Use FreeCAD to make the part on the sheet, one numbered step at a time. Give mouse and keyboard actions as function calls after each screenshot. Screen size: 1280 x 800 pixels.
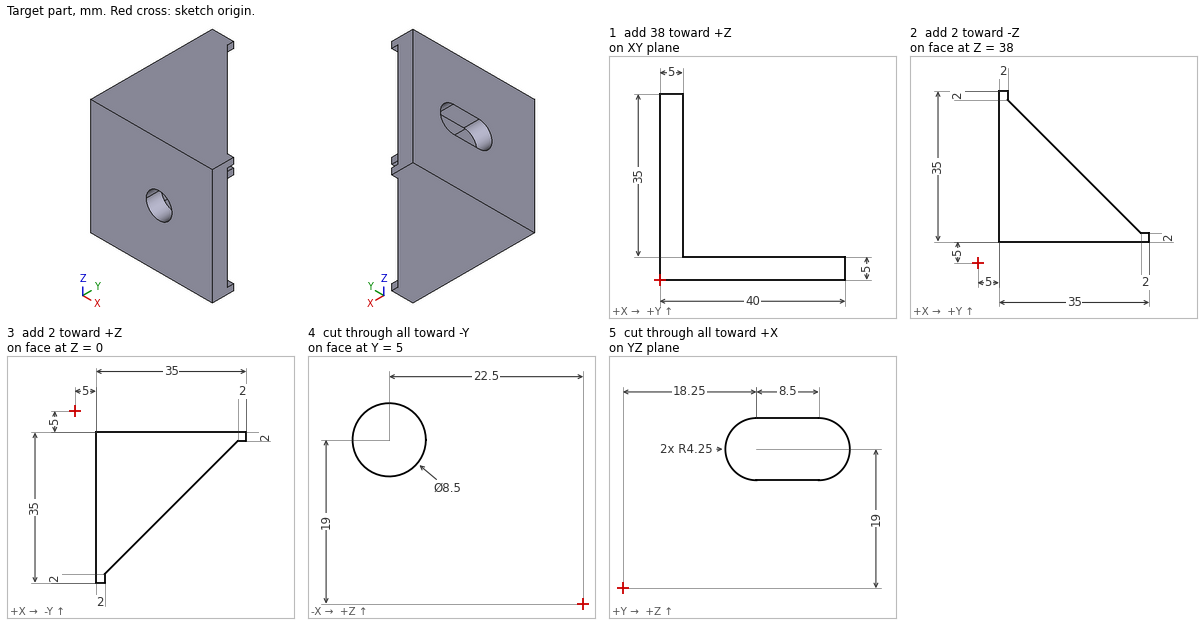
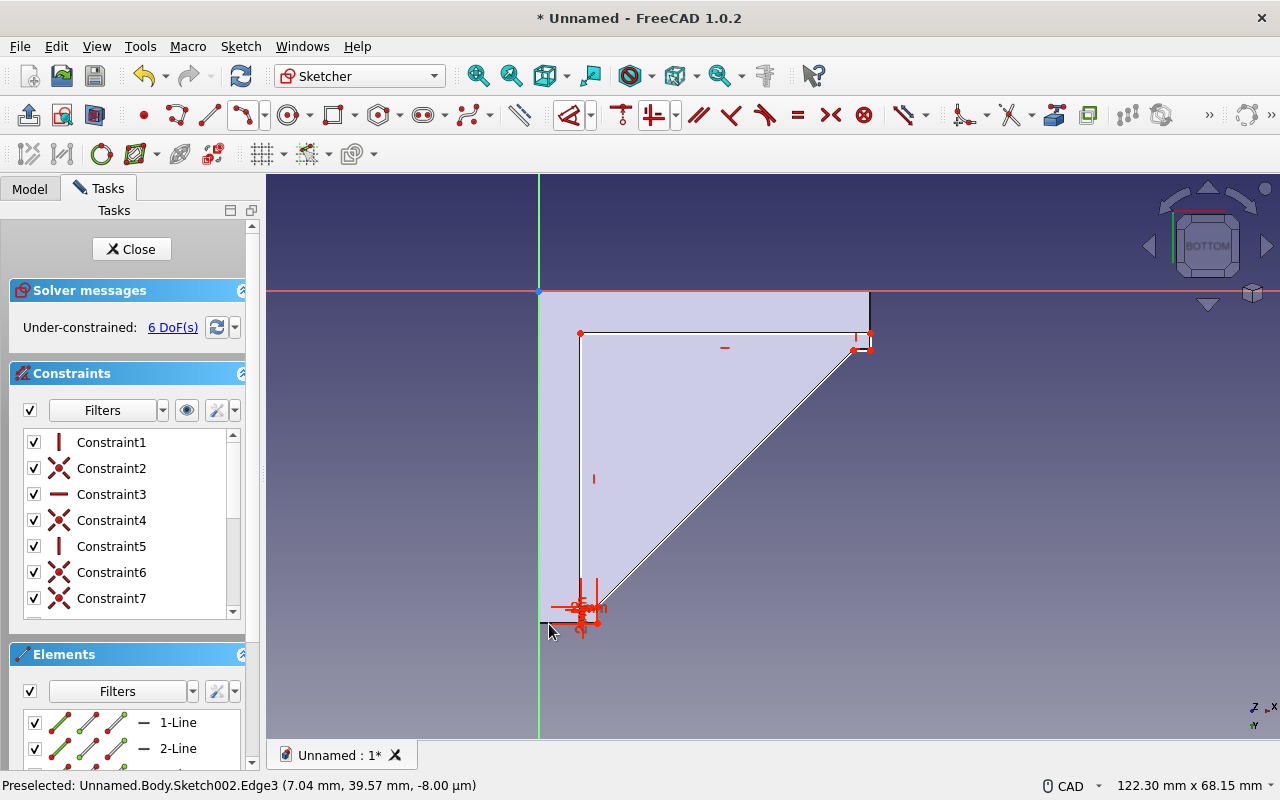
scroll(859, 351, up, 5)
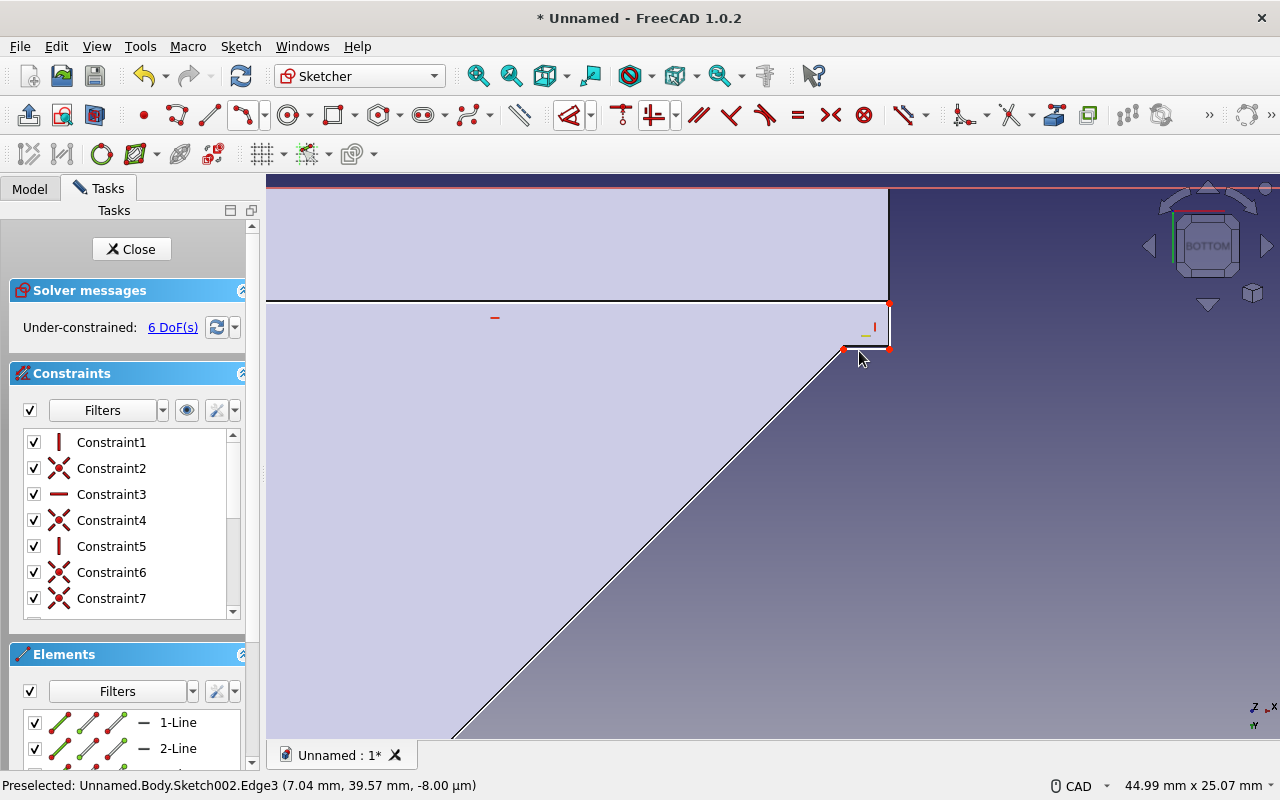
click(857, 349)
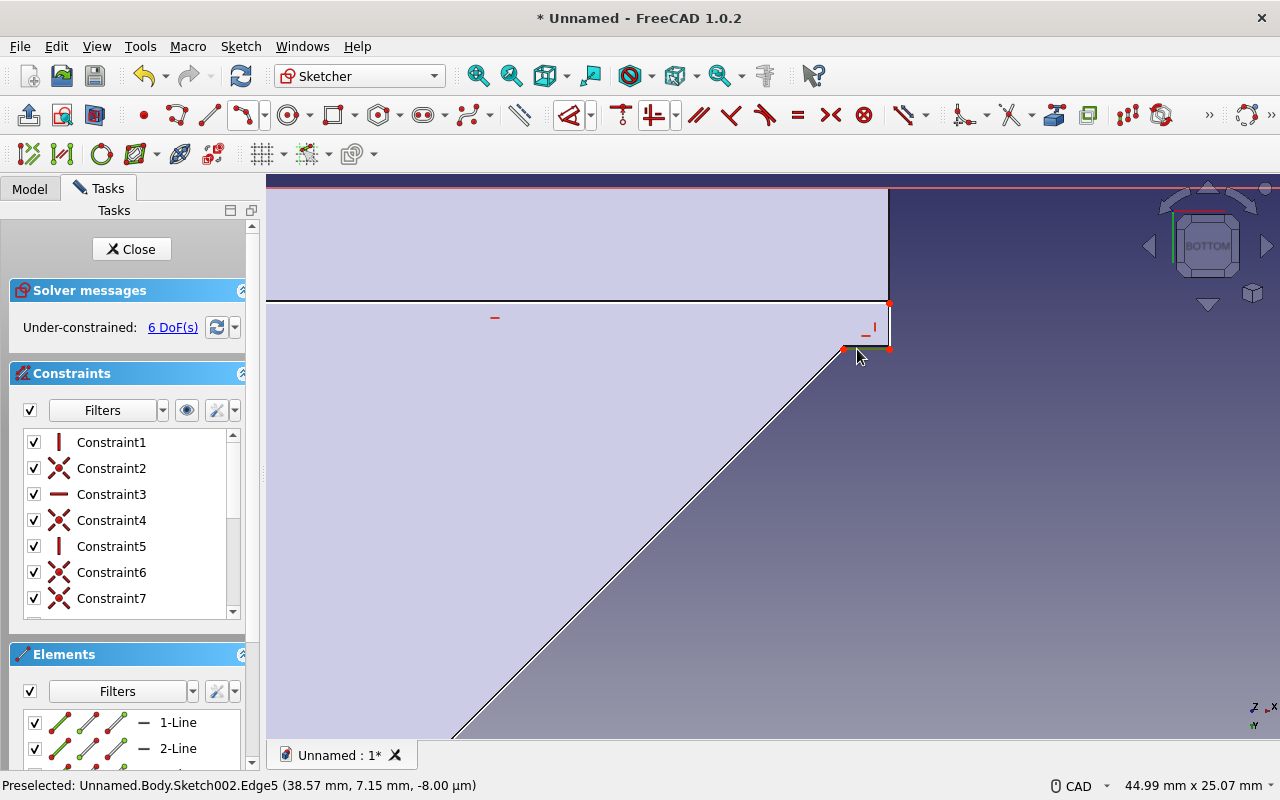
key(l)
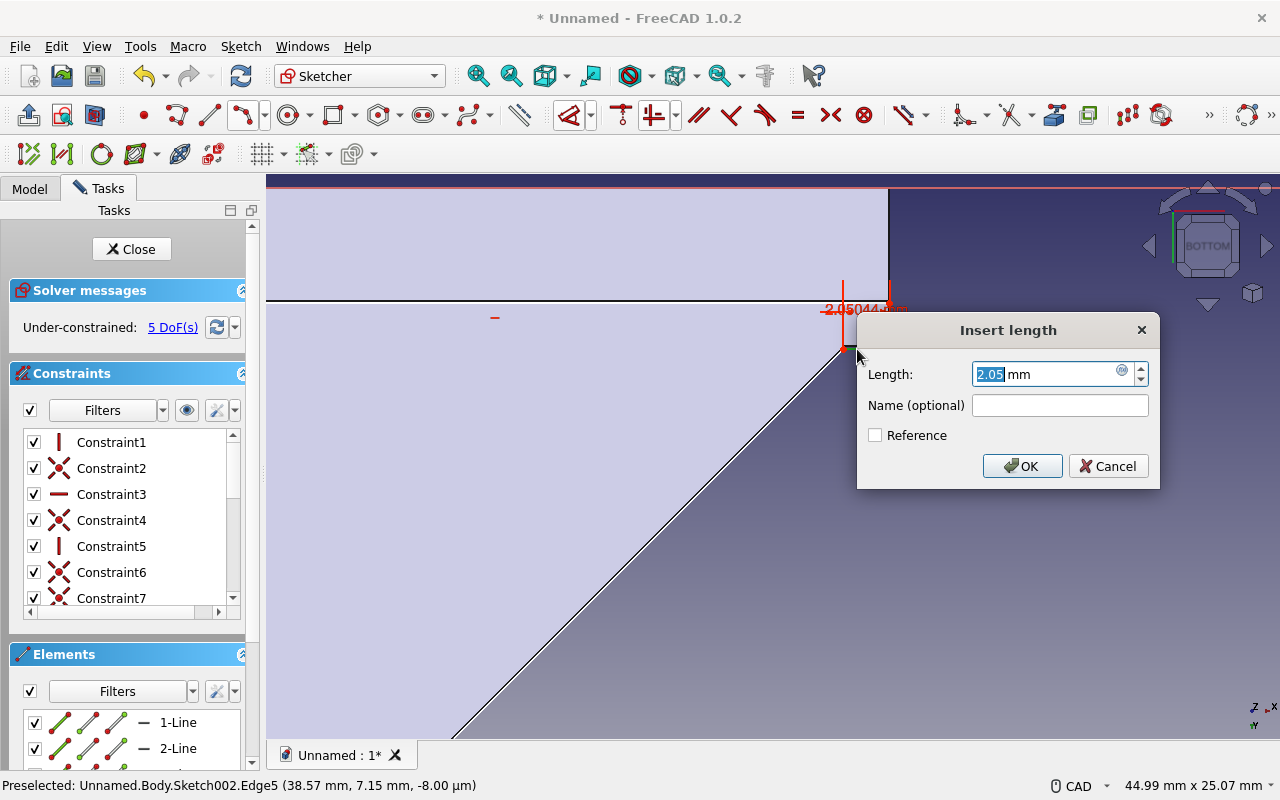
text(2)
key(Return)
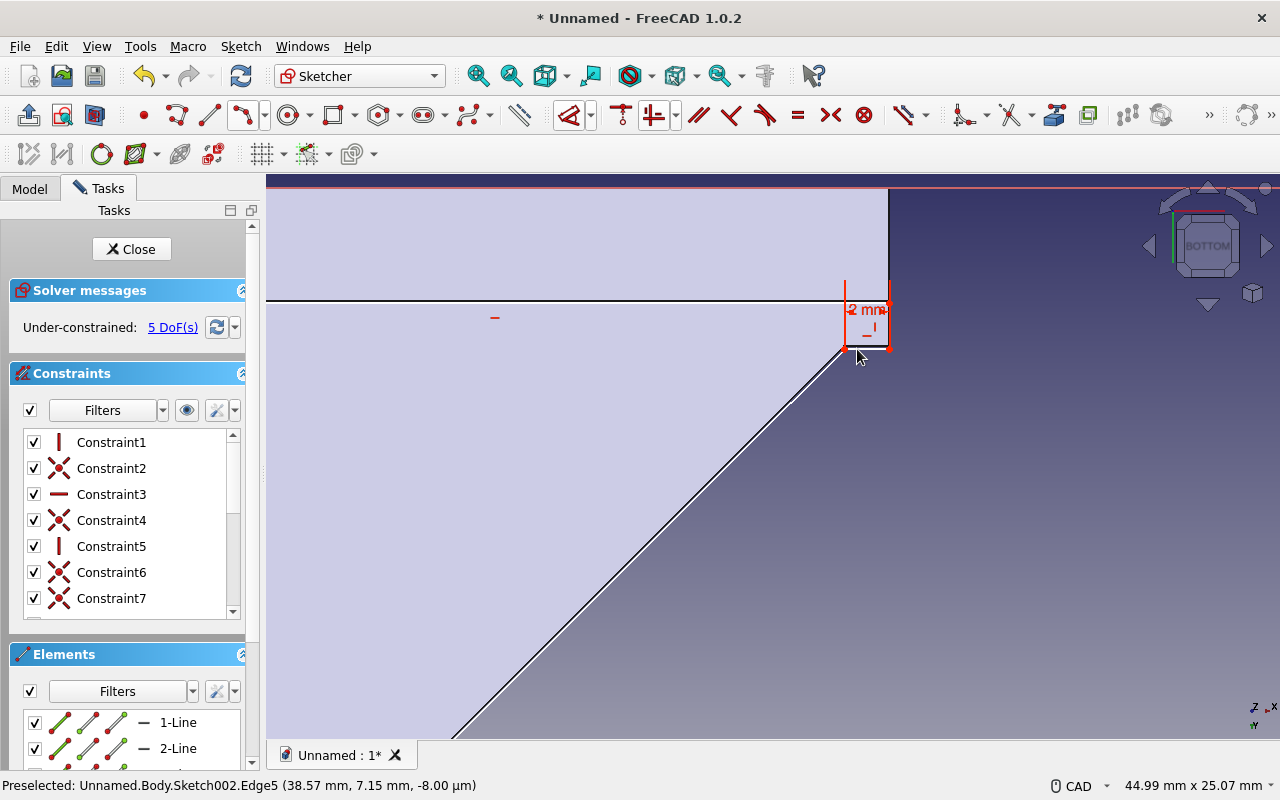
click(890, 336)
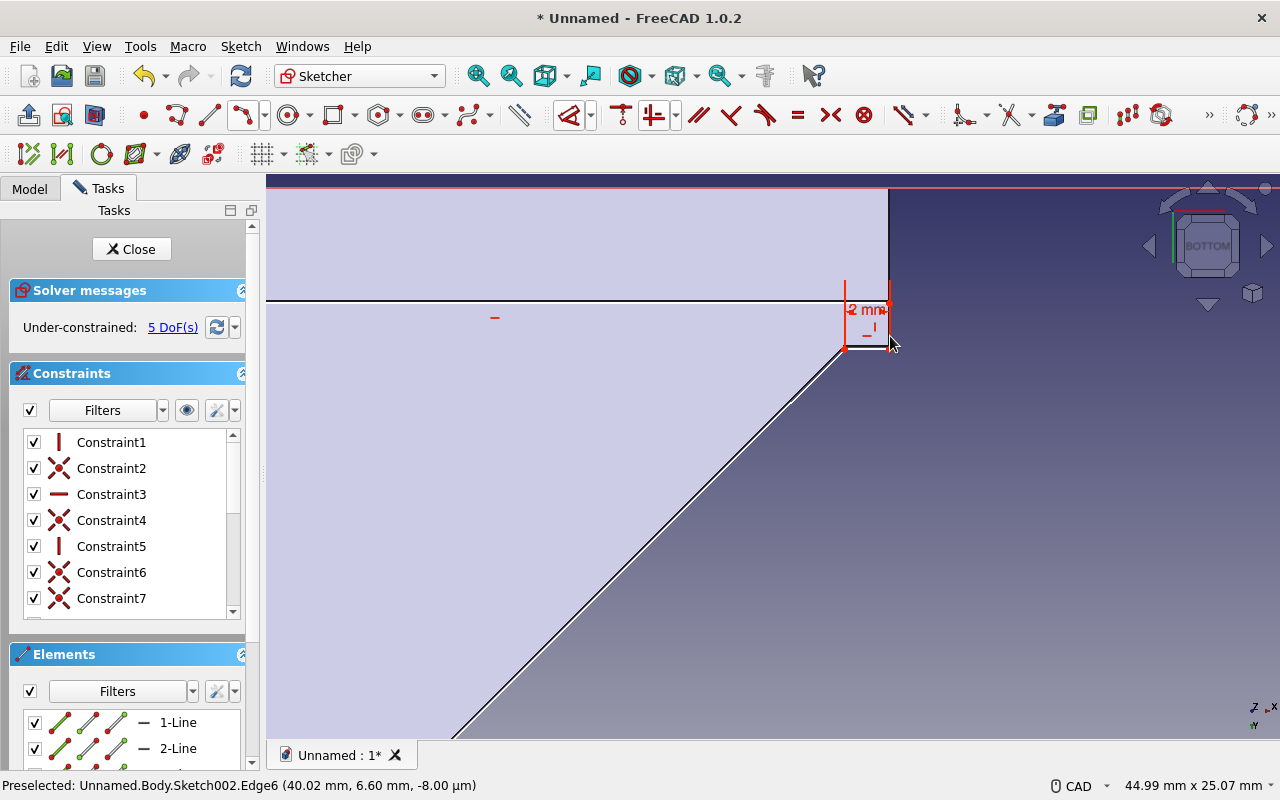
click(590, 116)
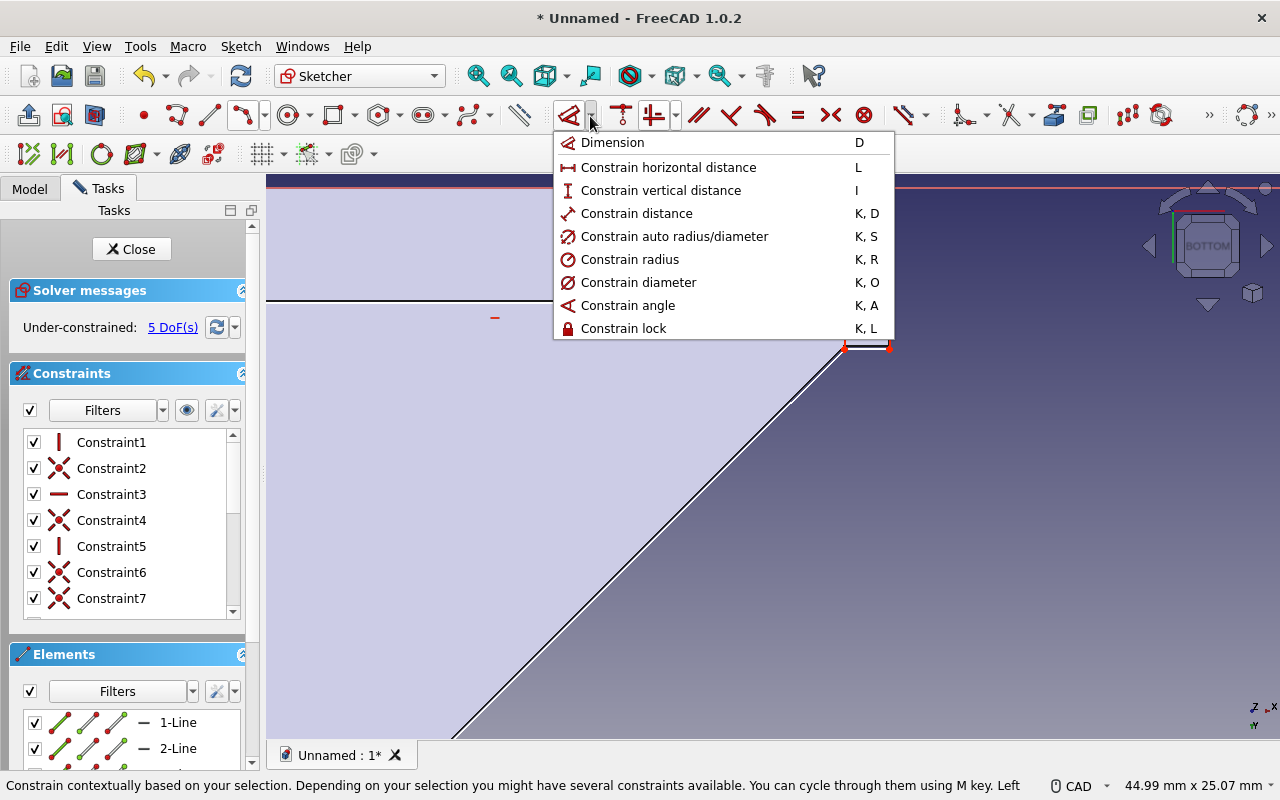
click(724, 190)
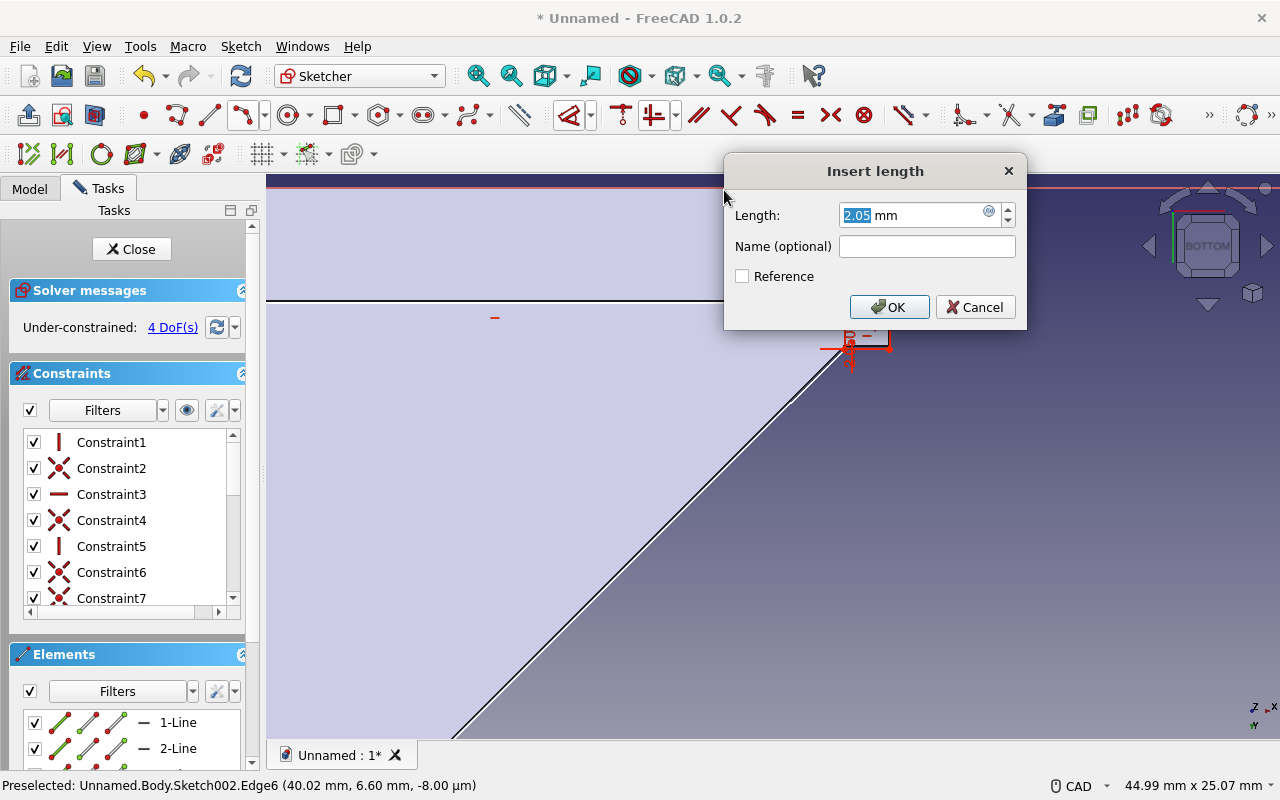
text(2)
key(Return)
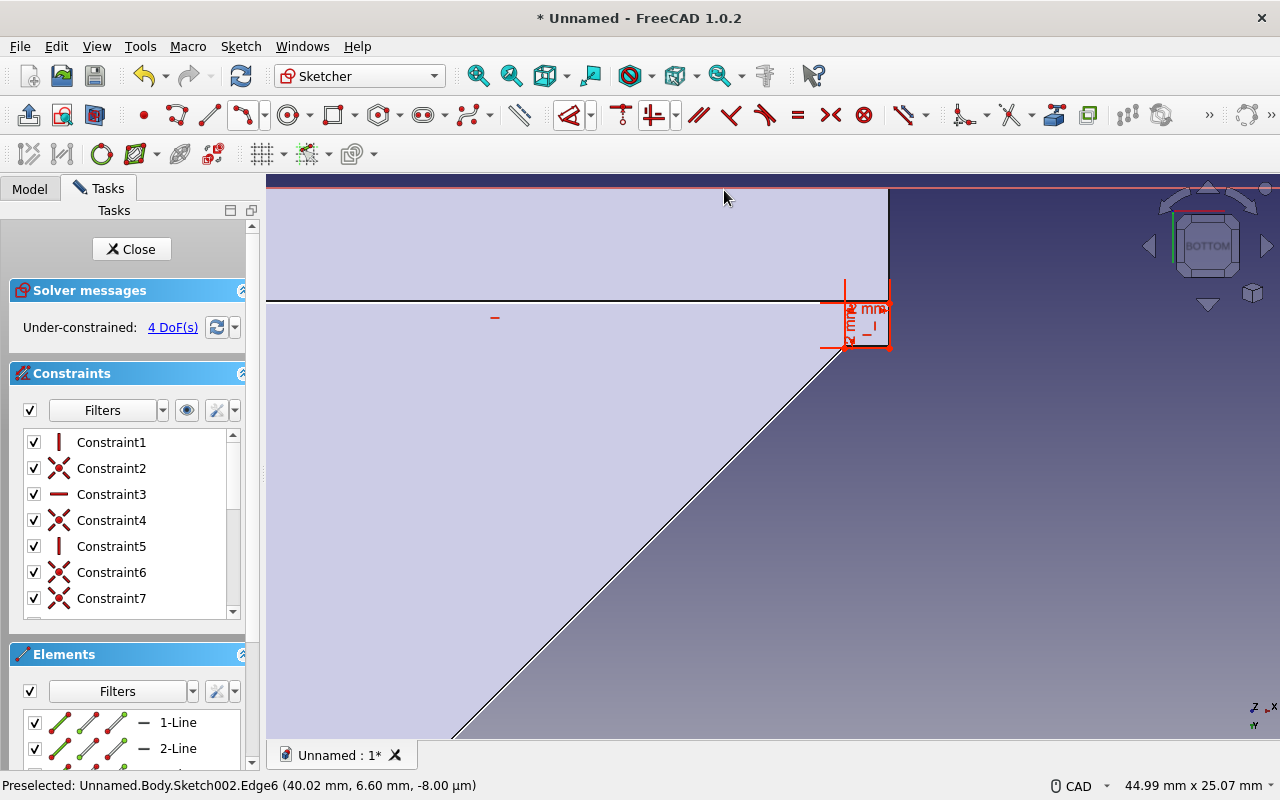
scroll(859, 350, down, 5)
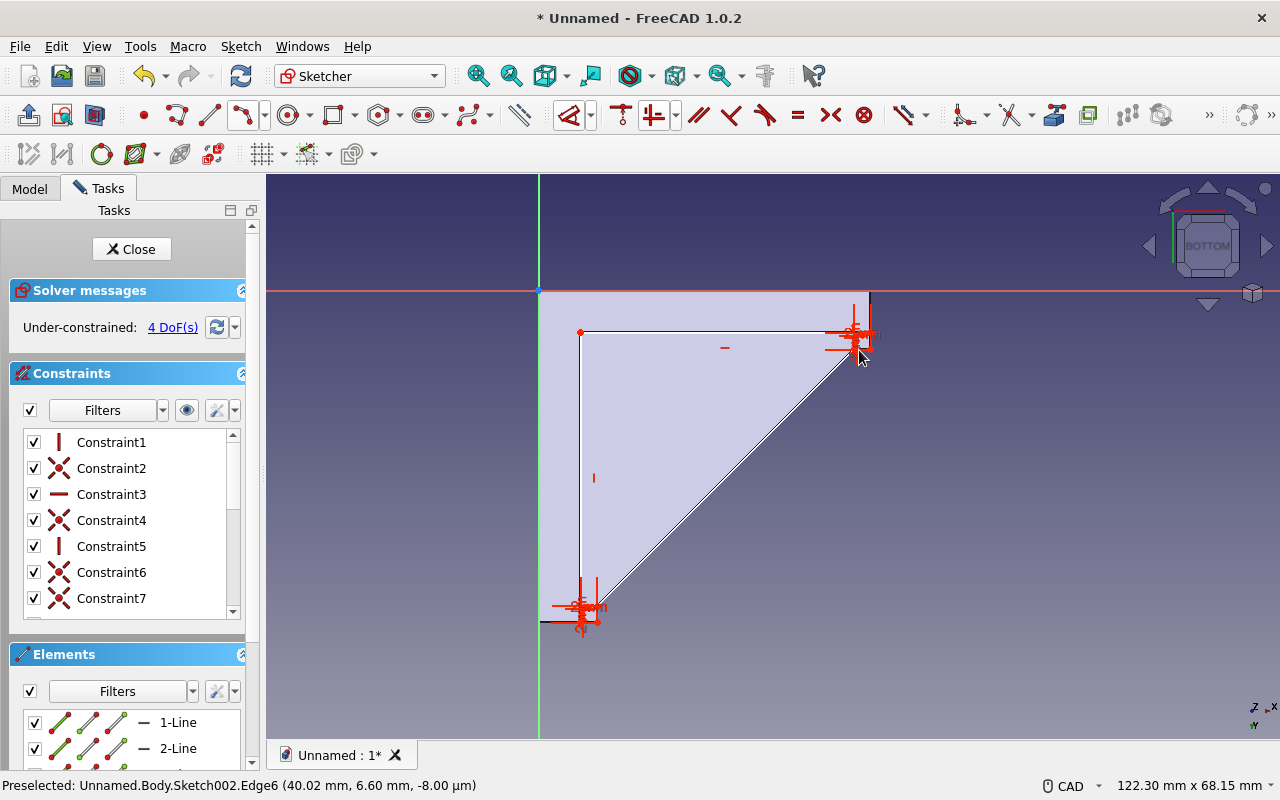
click(581, 420)